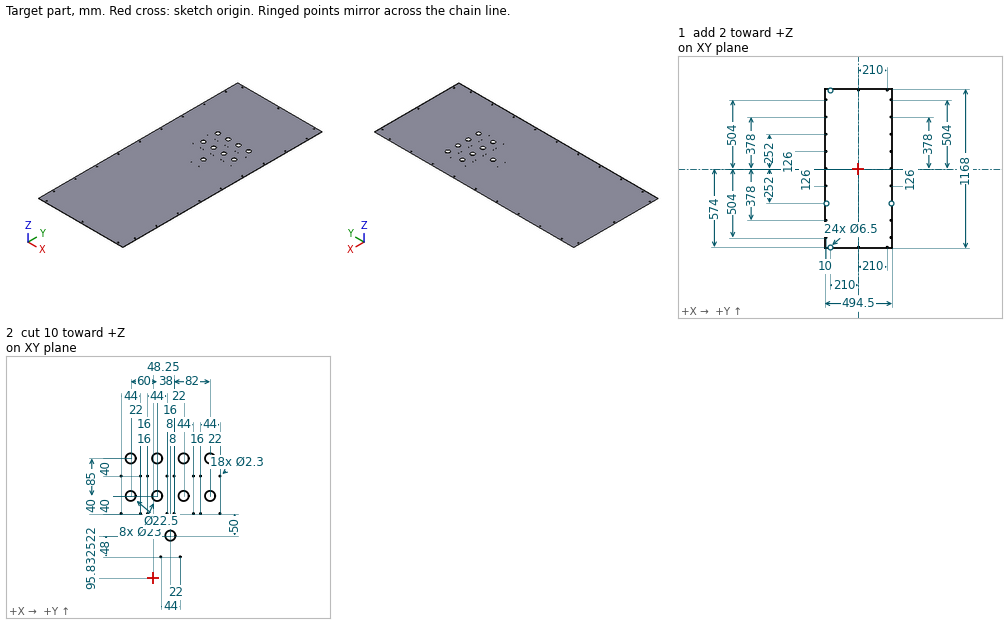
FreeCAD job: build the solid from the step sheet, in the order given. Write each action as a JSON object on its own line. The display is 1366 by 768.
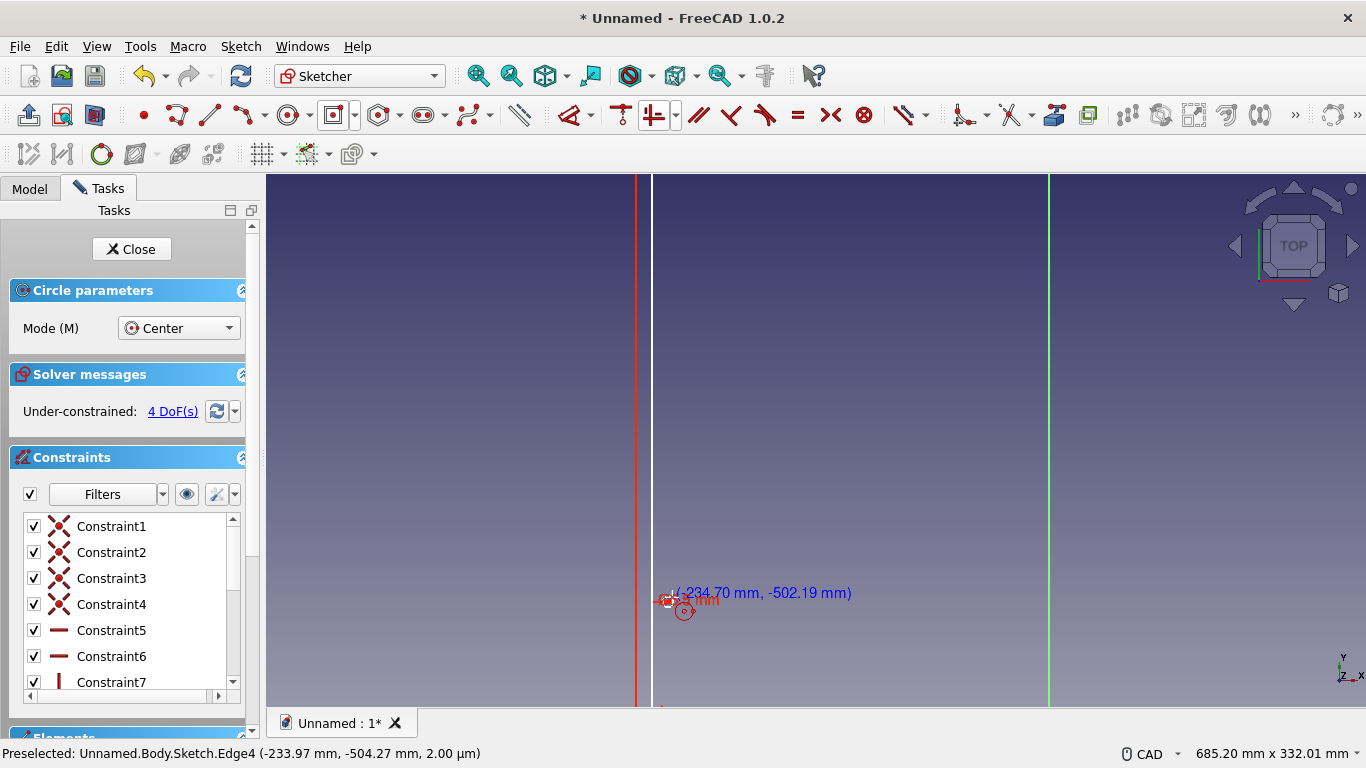
{"action": "scroll", "coordinate": [668, 399], "scroll_direction": "up", "scroll_amount": 8}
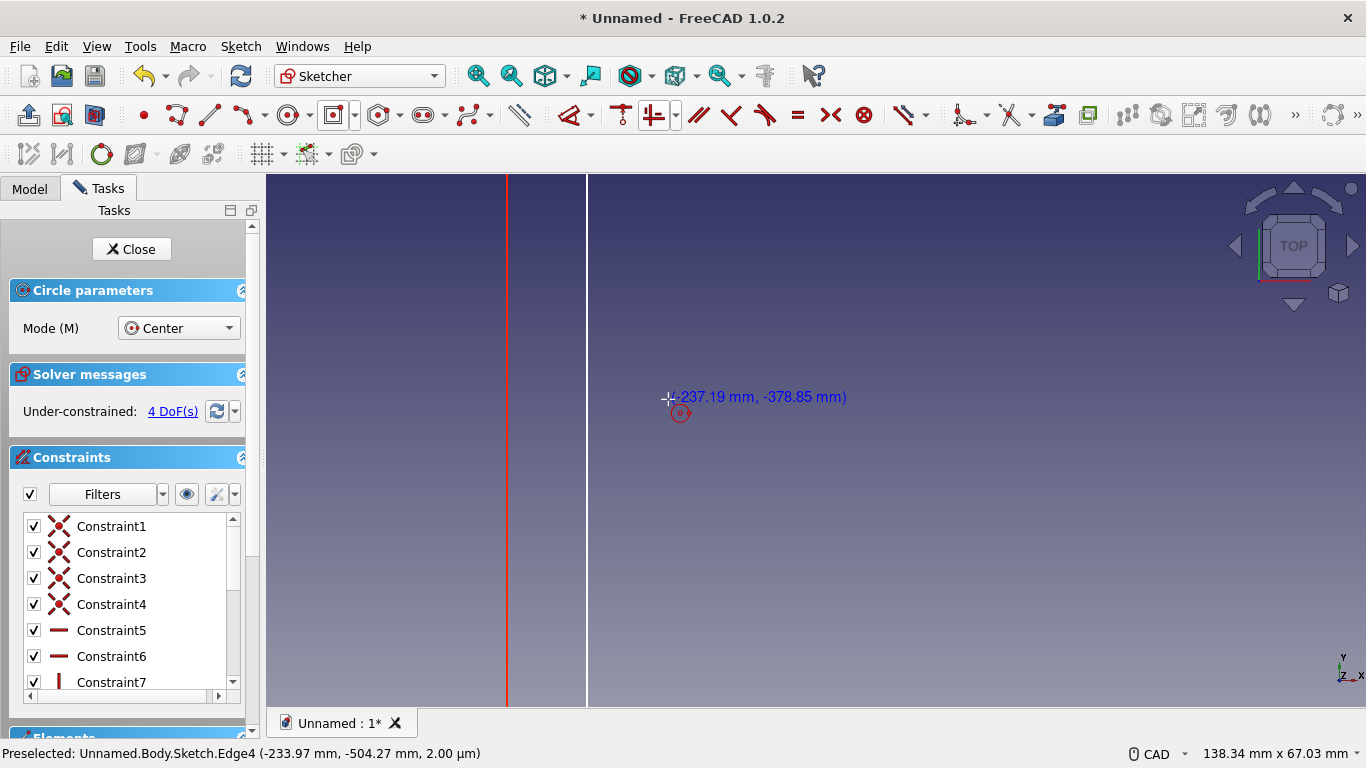
{"action": "scroll", "coordinate": [671, 570], "scroll_direction": "down", "scroll_amount": 16}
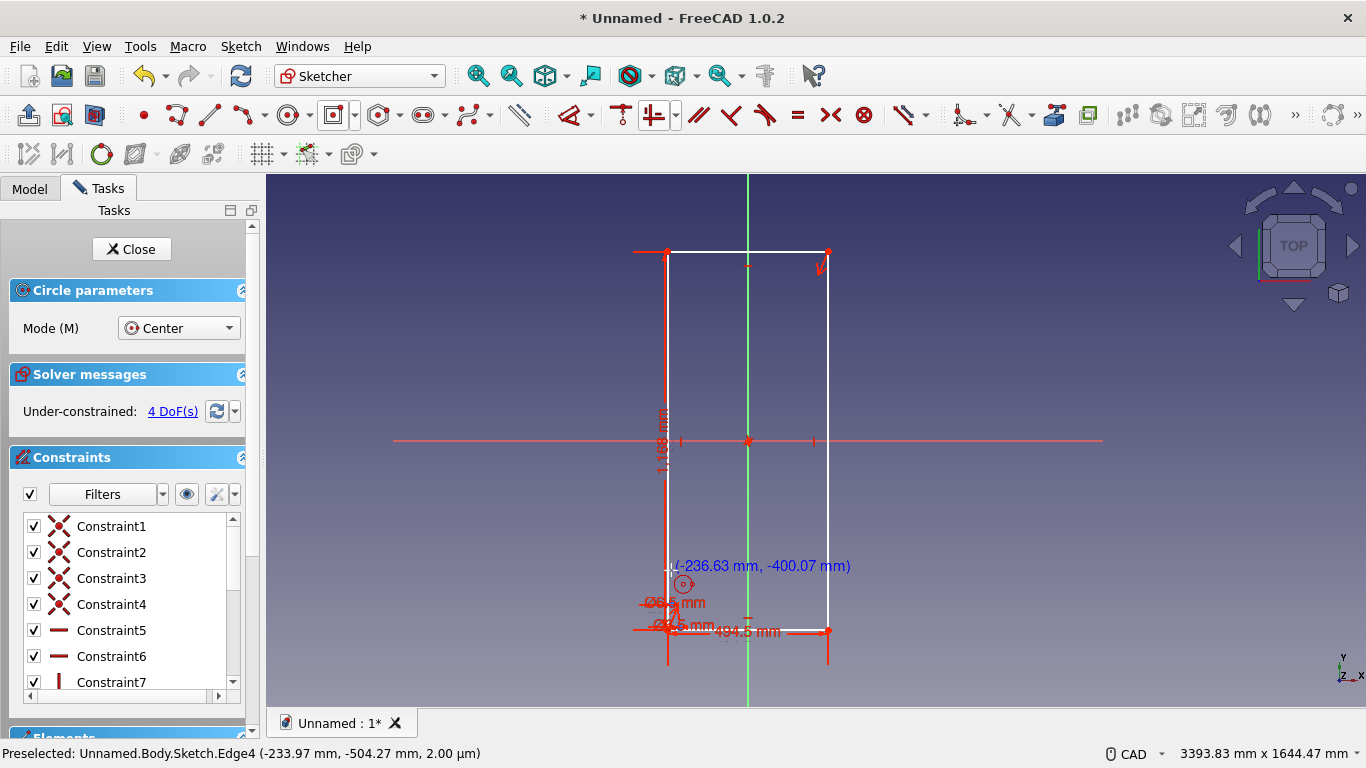
{"action": "scroll", "coordinate": [671, 564], "scroll_direction": "up", "scroll_amount": 8}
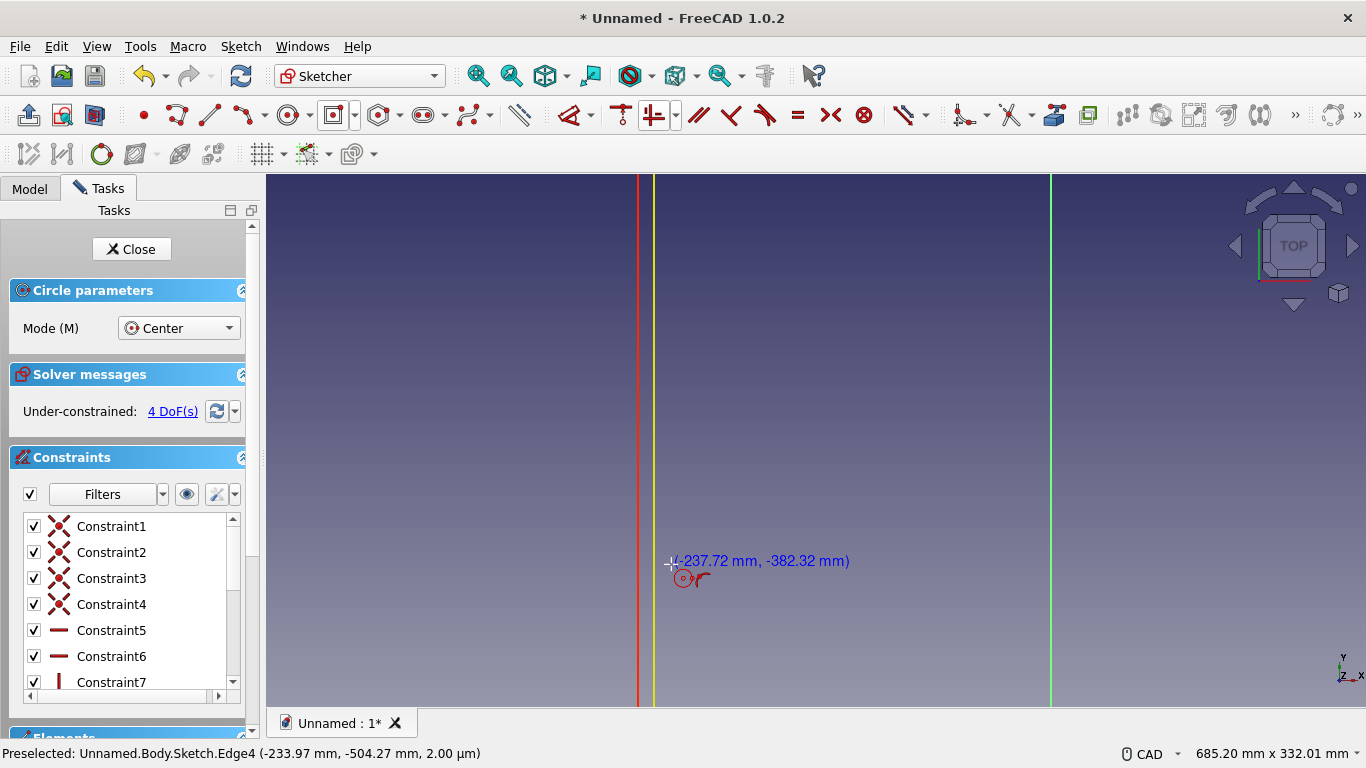
{"action": "left_click", "coordinate": [670, 559]}
{"action": "mouse_move", "coordinate": [674, 555]}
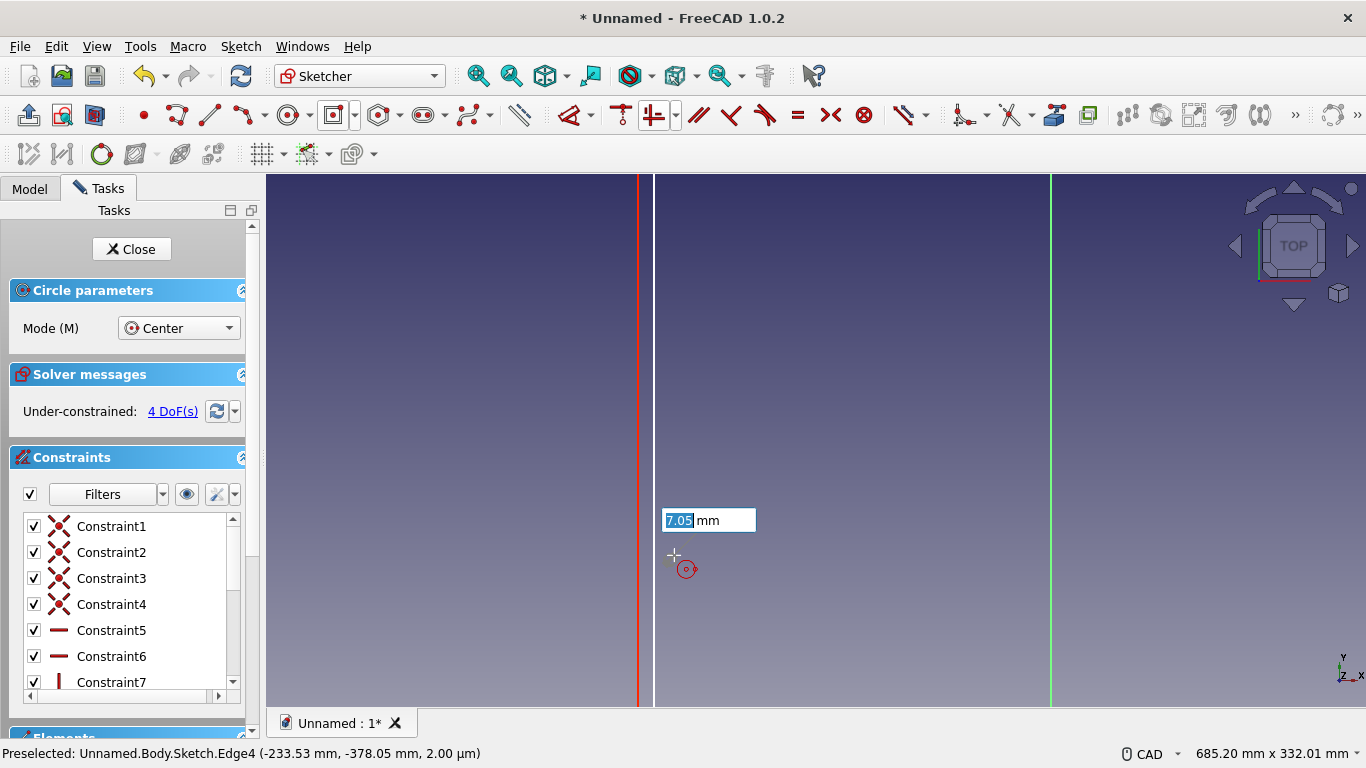
{"action": "type", "text": "6.5"}
{"action": "key", "text": "Return"}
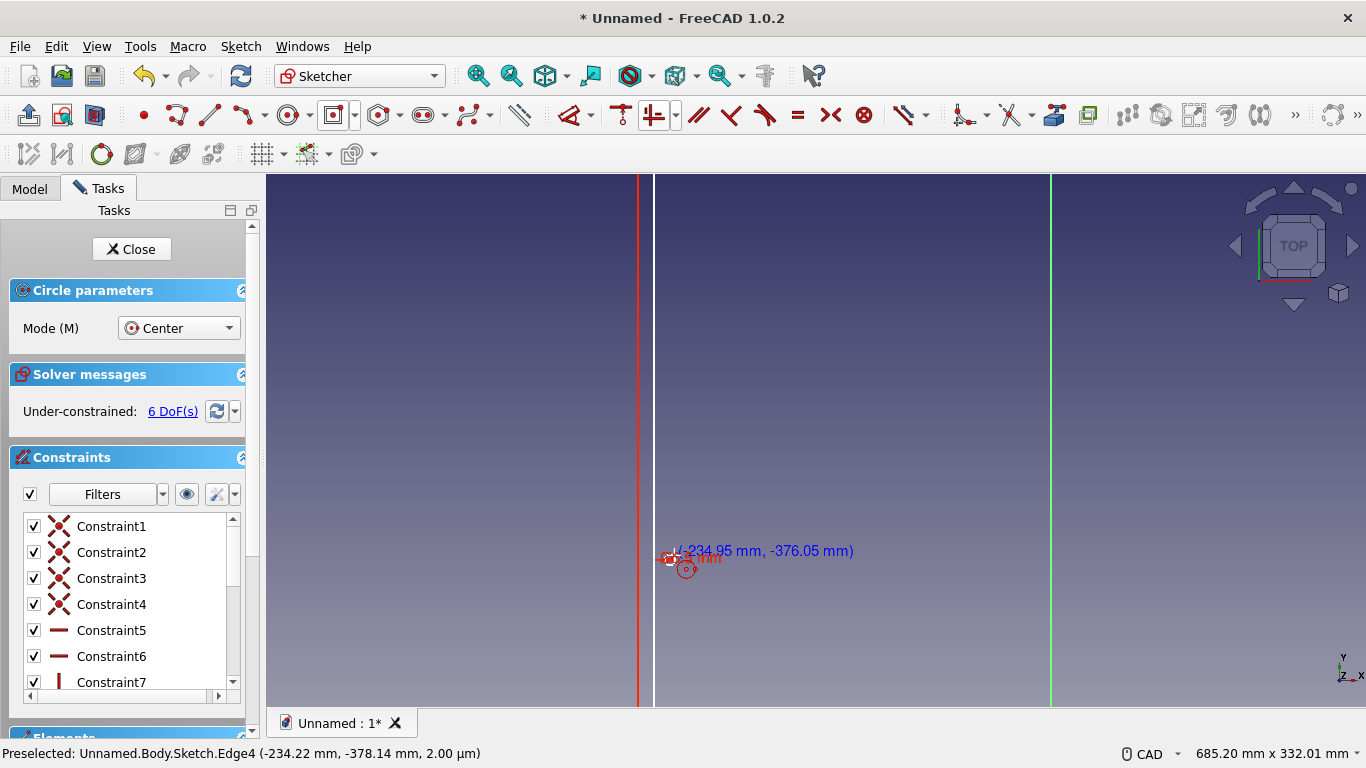
{"action": "scroll", "coordinate": [670, 357], "scroll_direction": "up", "scroll_amount": 8}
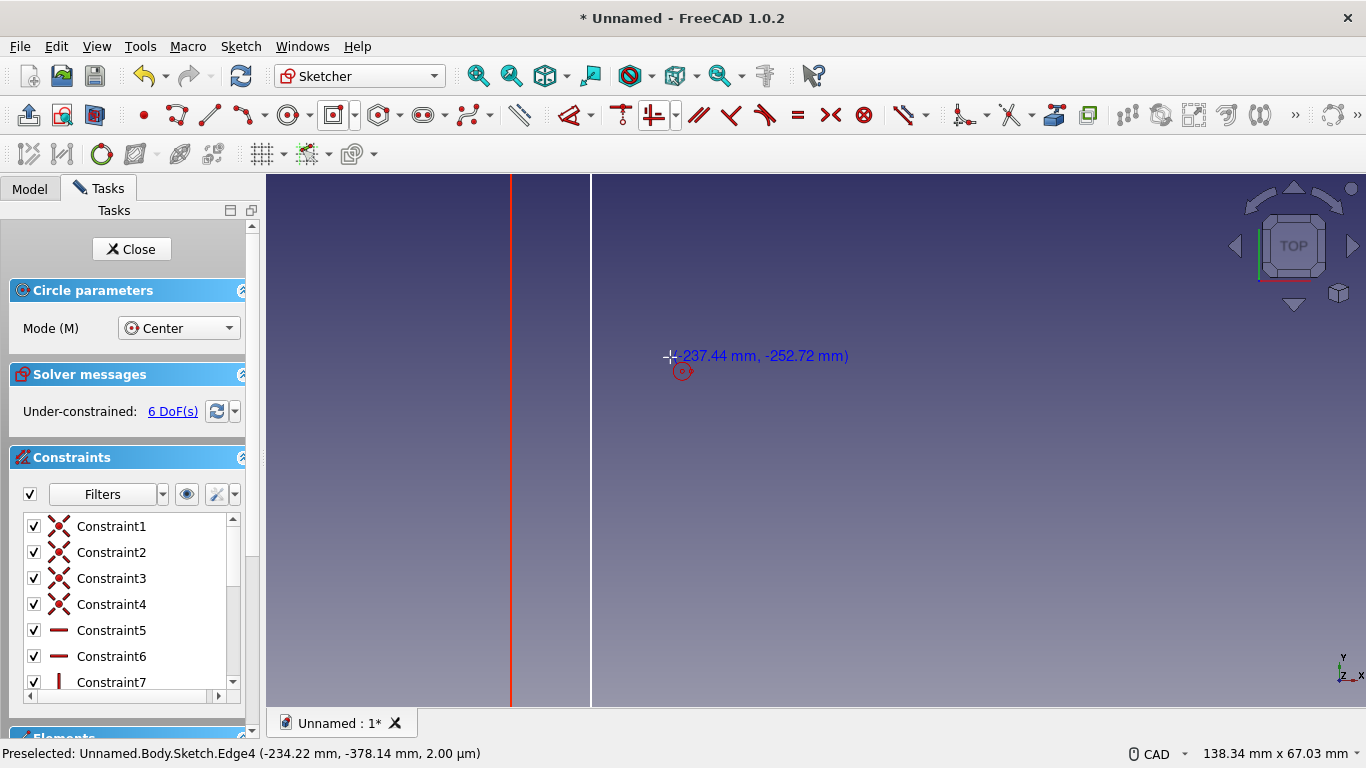
{"action": "scroll", "coordinate": [671, 529], "scroll_direction": "down", "scroll_amount": 16}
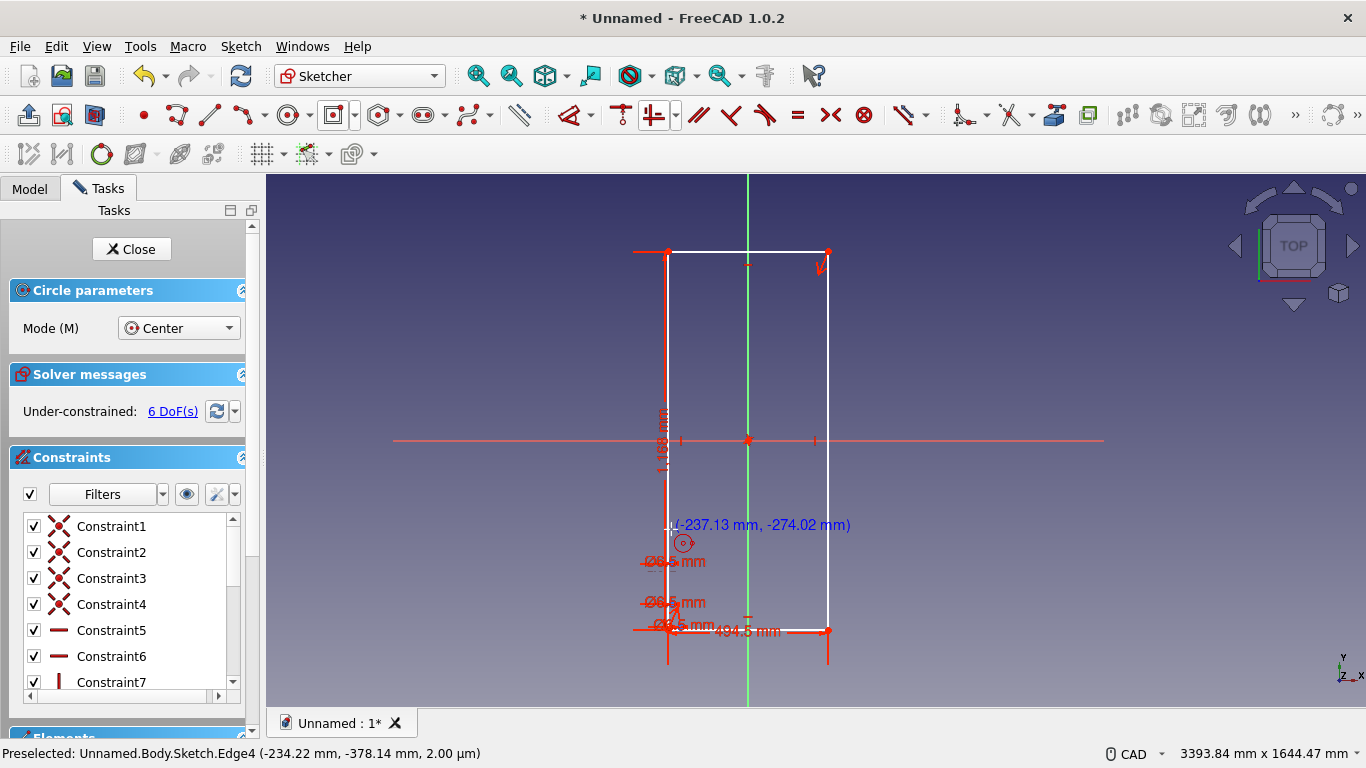
{"action": "scroll", "coordinate": [671, 523], "scroll_direction": "up", "scroll_amount": 8}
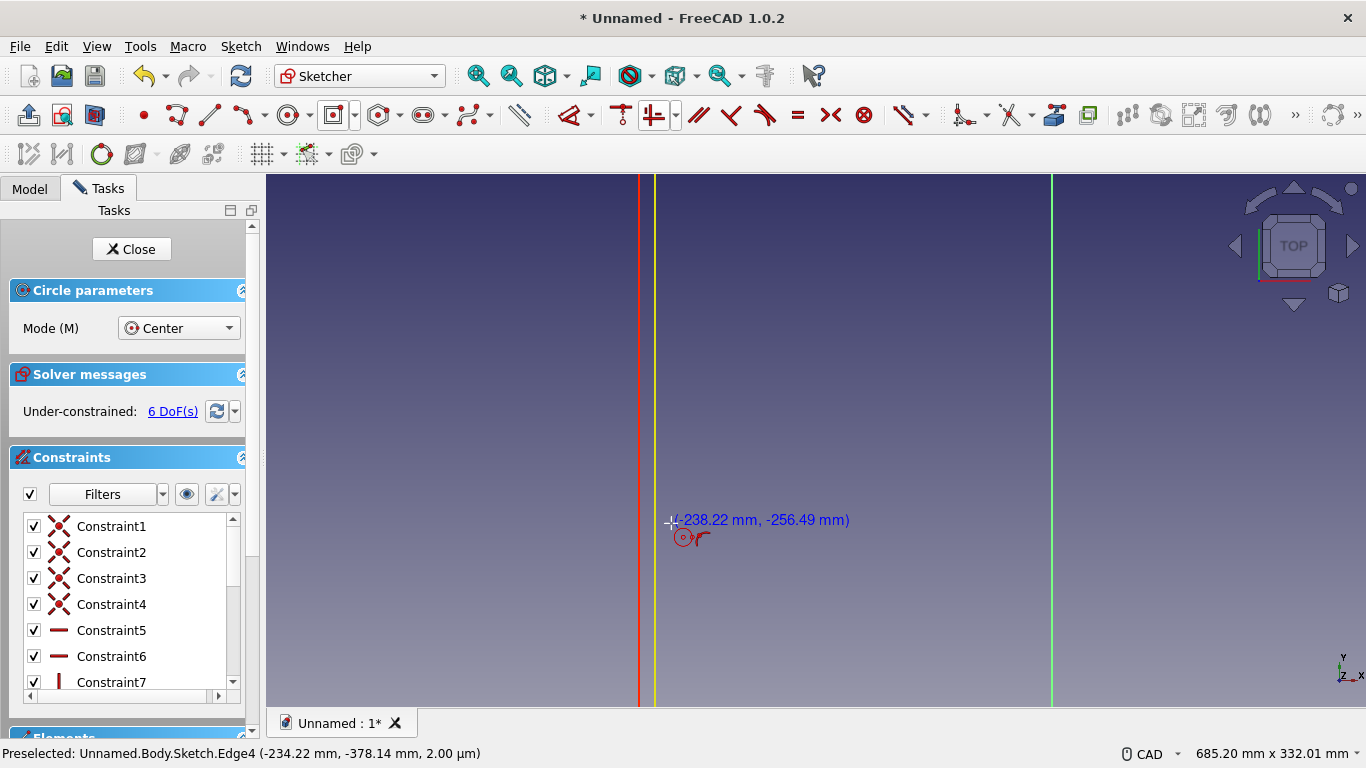
{"action": "left_click", "coordinate": [671, 518]}
{"action": "mouse_move", "coordinate": [675, 514]}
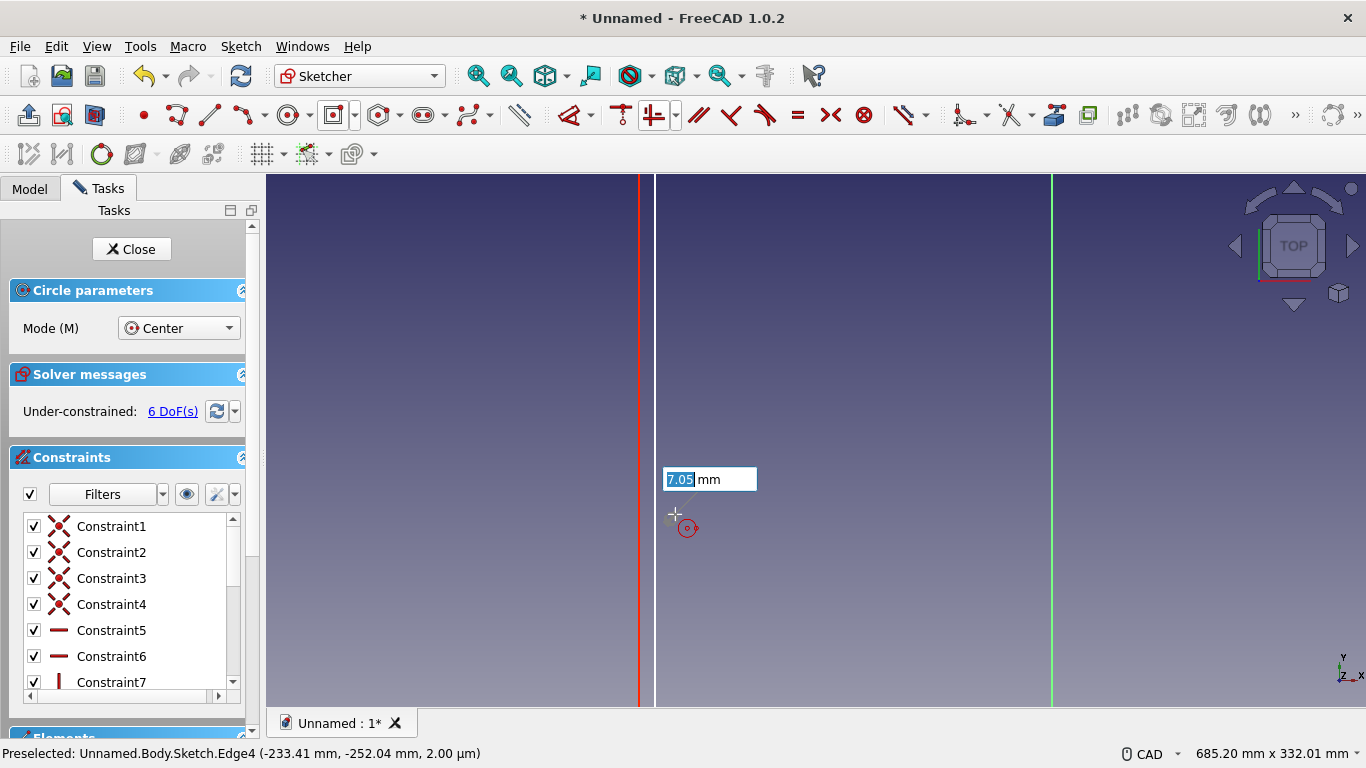
{"action": "type", "text": "6.5"}
{"action": "key", "text": "Return"}